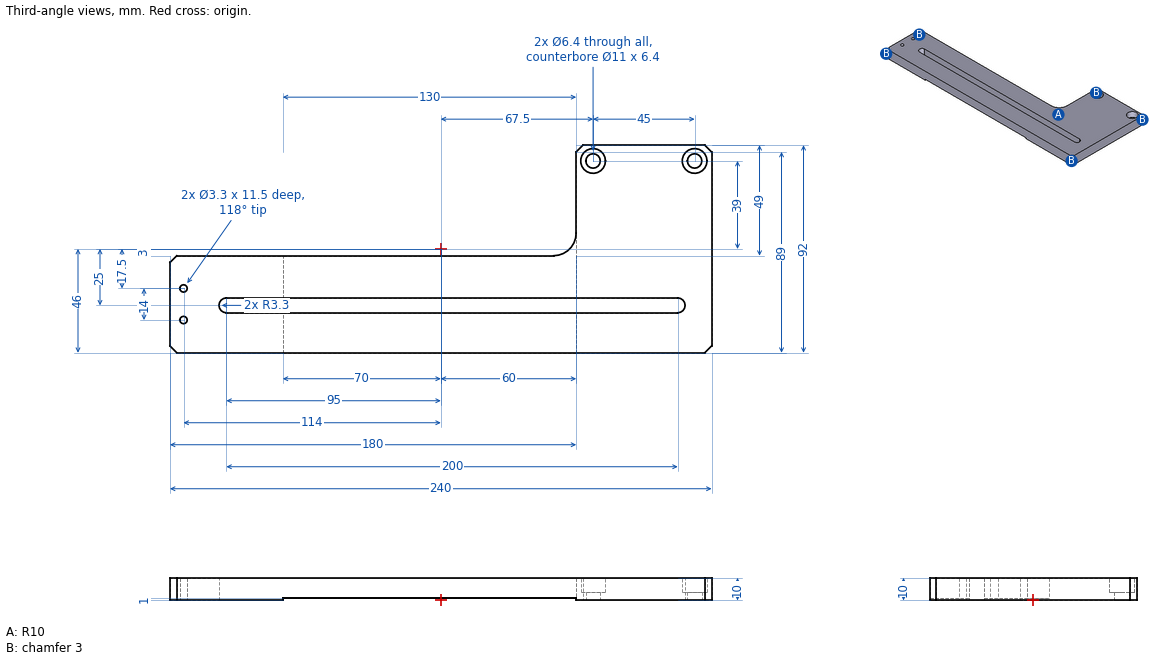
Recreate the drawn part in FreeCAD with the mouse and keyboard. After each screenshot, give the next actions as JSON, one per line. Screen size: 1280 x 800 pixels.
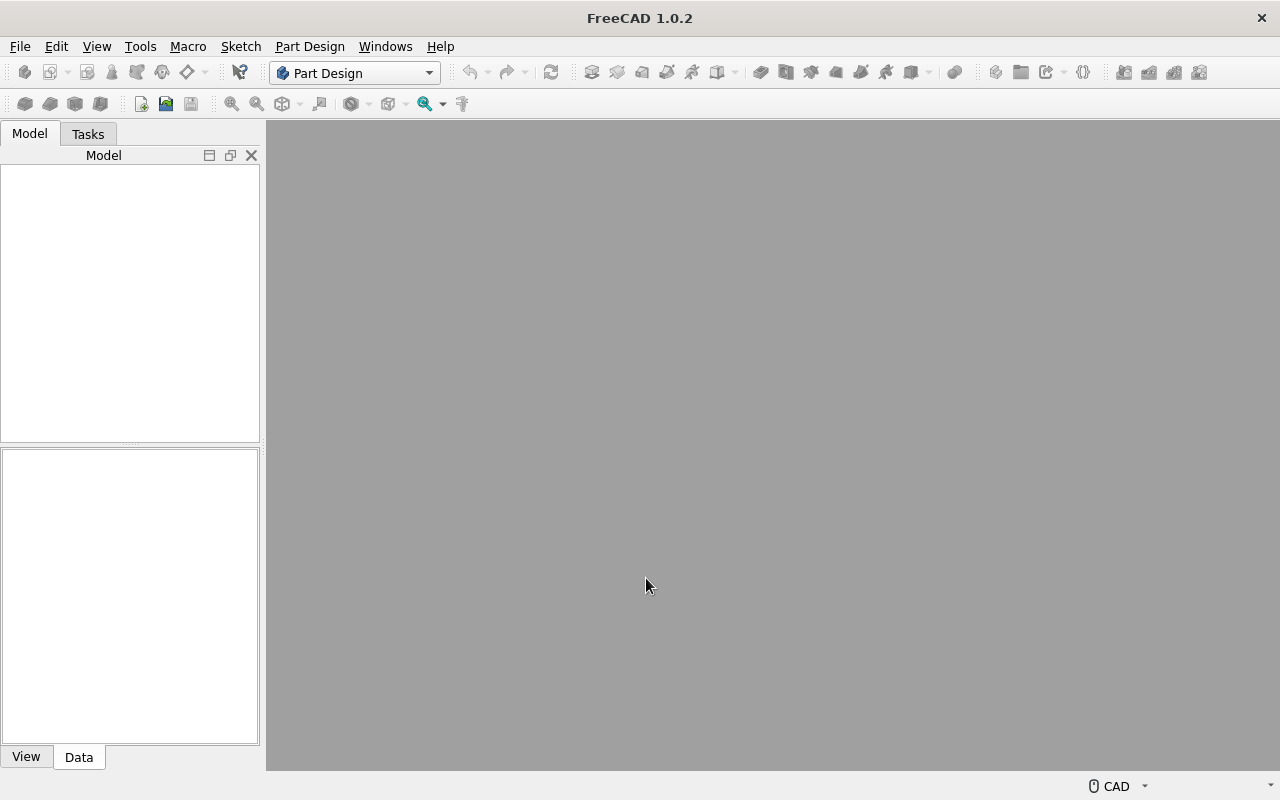
{"action": "left_click", "coordinate": [141, 104]}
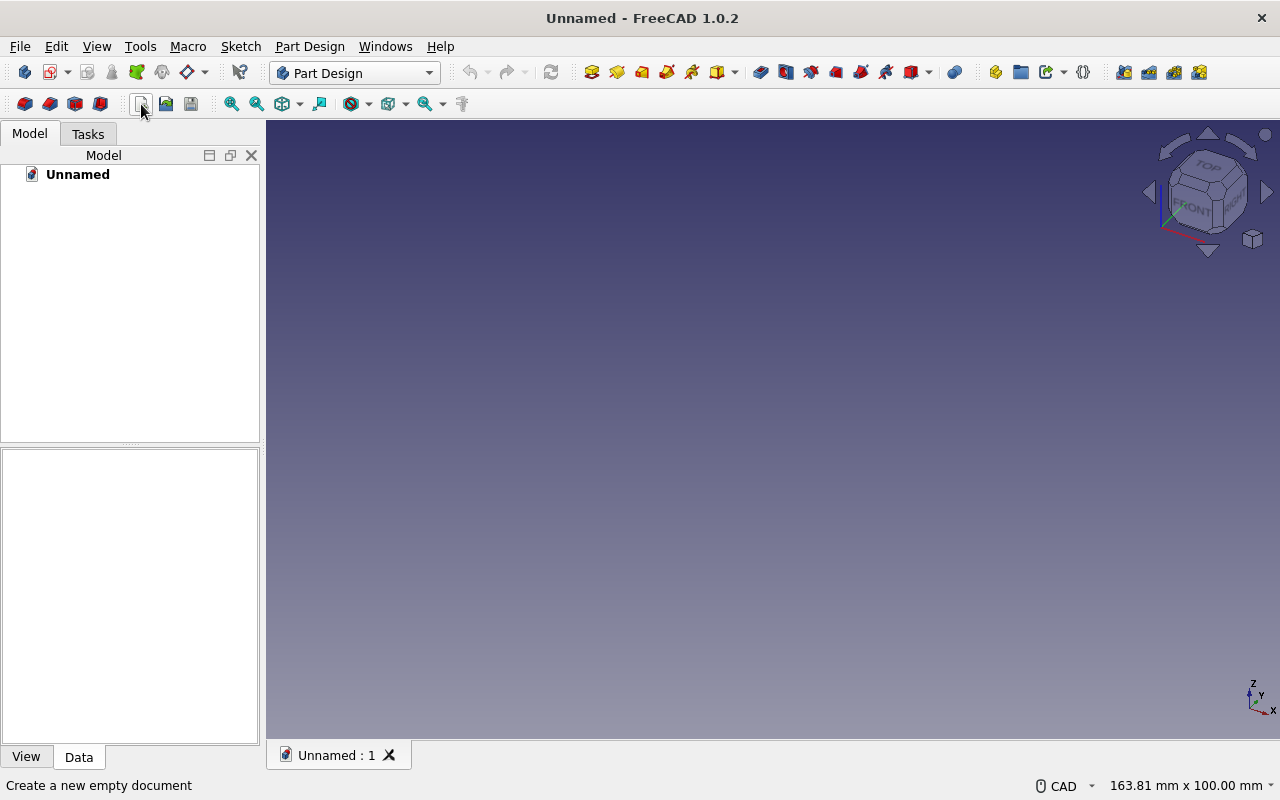
{"action": "left_click", "coordinate": [50, 72]}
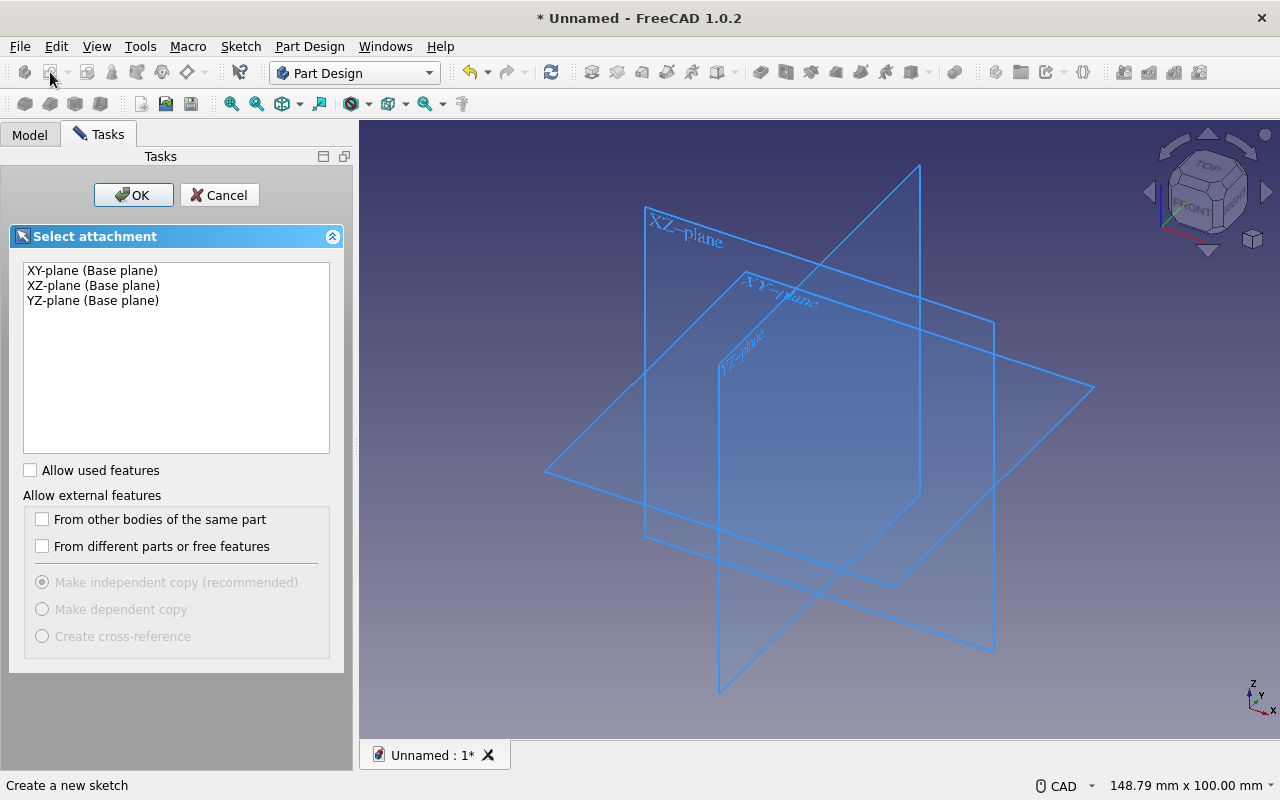
{"action": "left_click", "coordinate": [84, 270]}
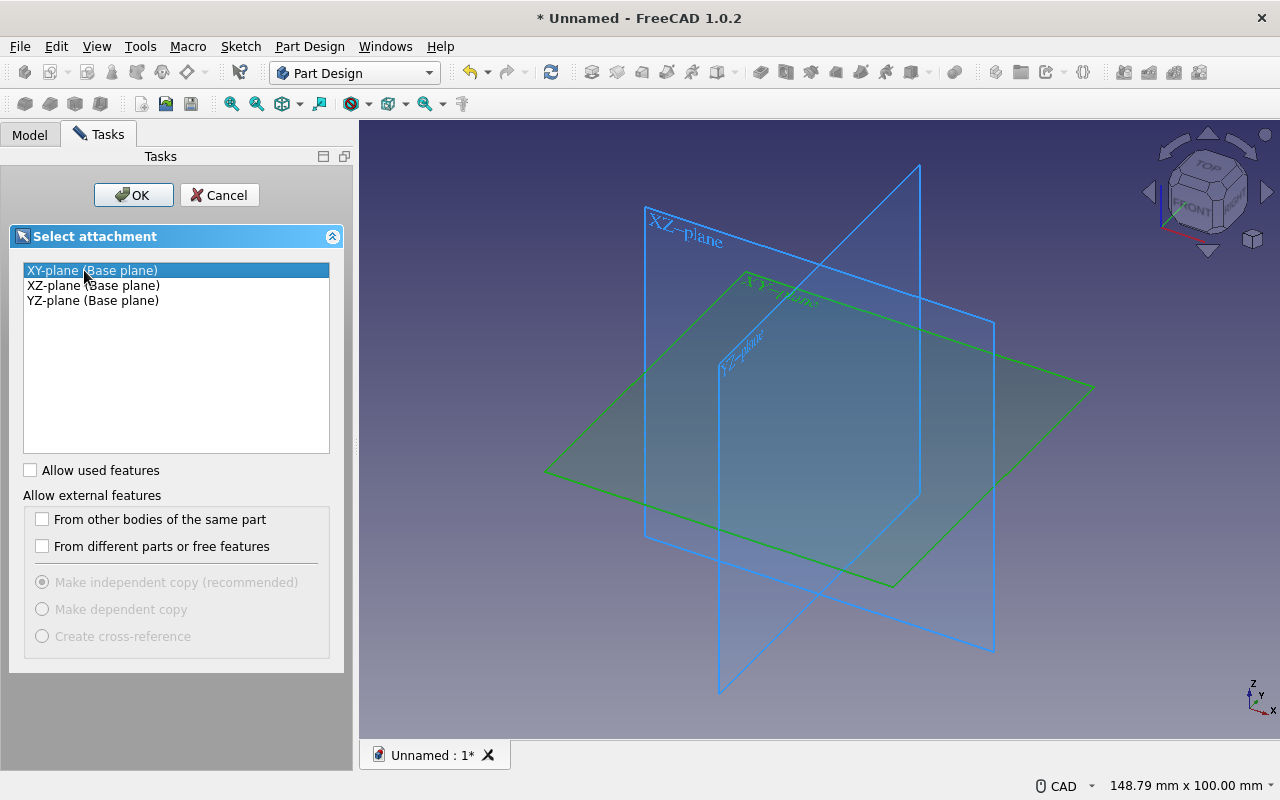
{"action": "left_click", "coordinate": [134, 195]}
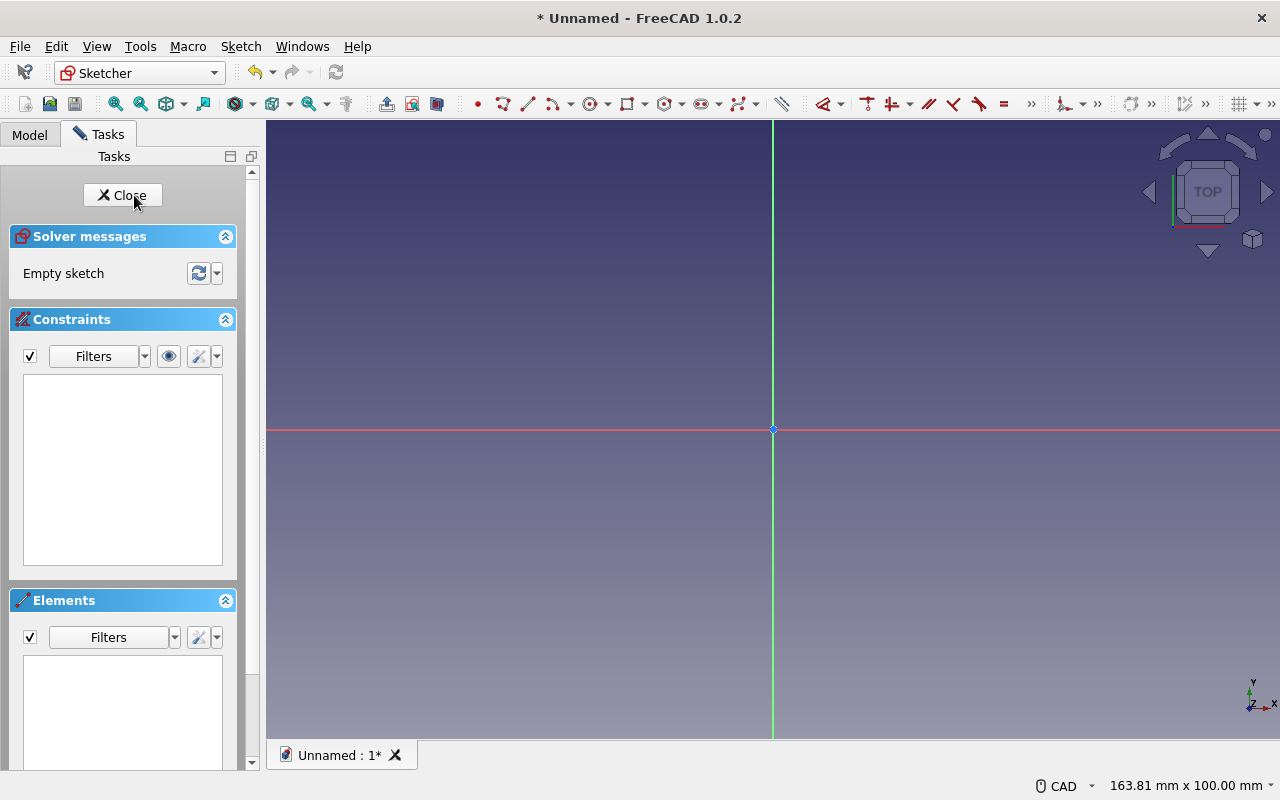
{"action": "scroll", "coordinate": [665, 430], "scroll_direction": "down", "scroll_amount": 5}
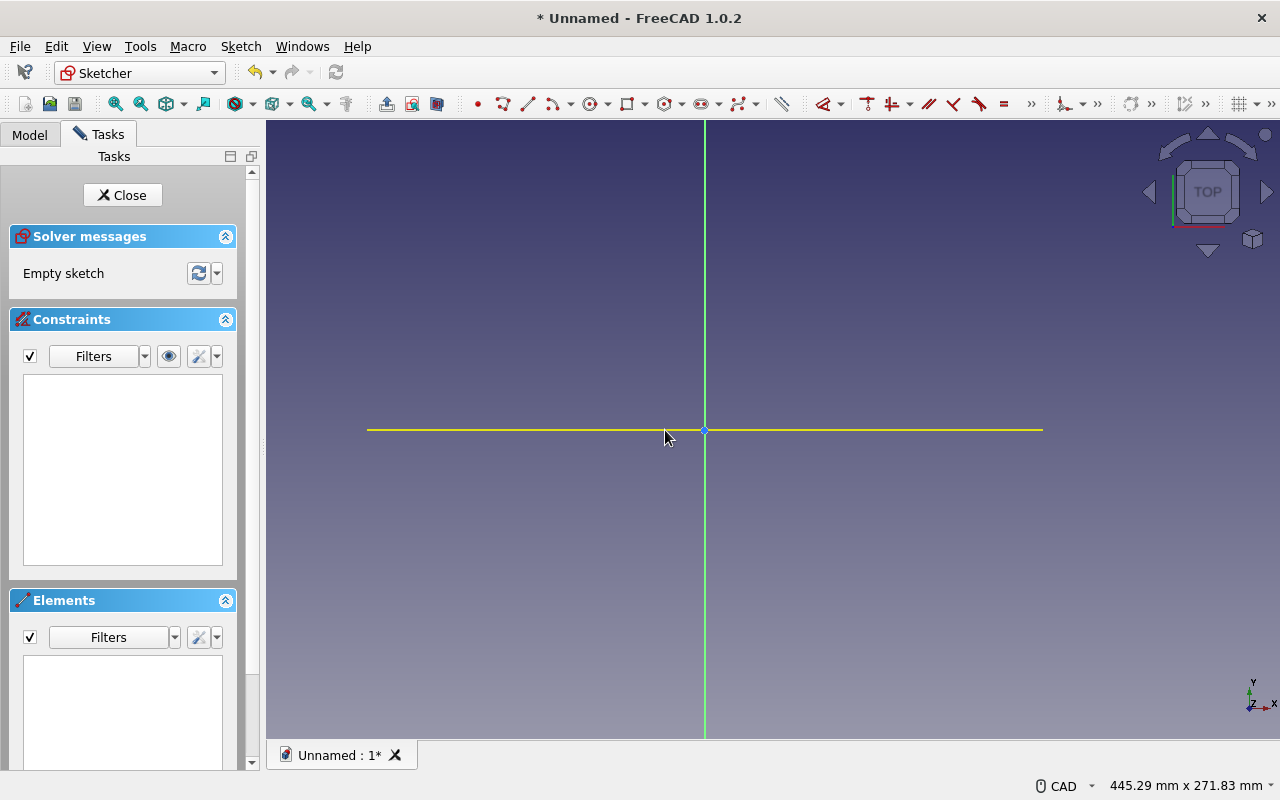
{"action": "key", "text": "g v"}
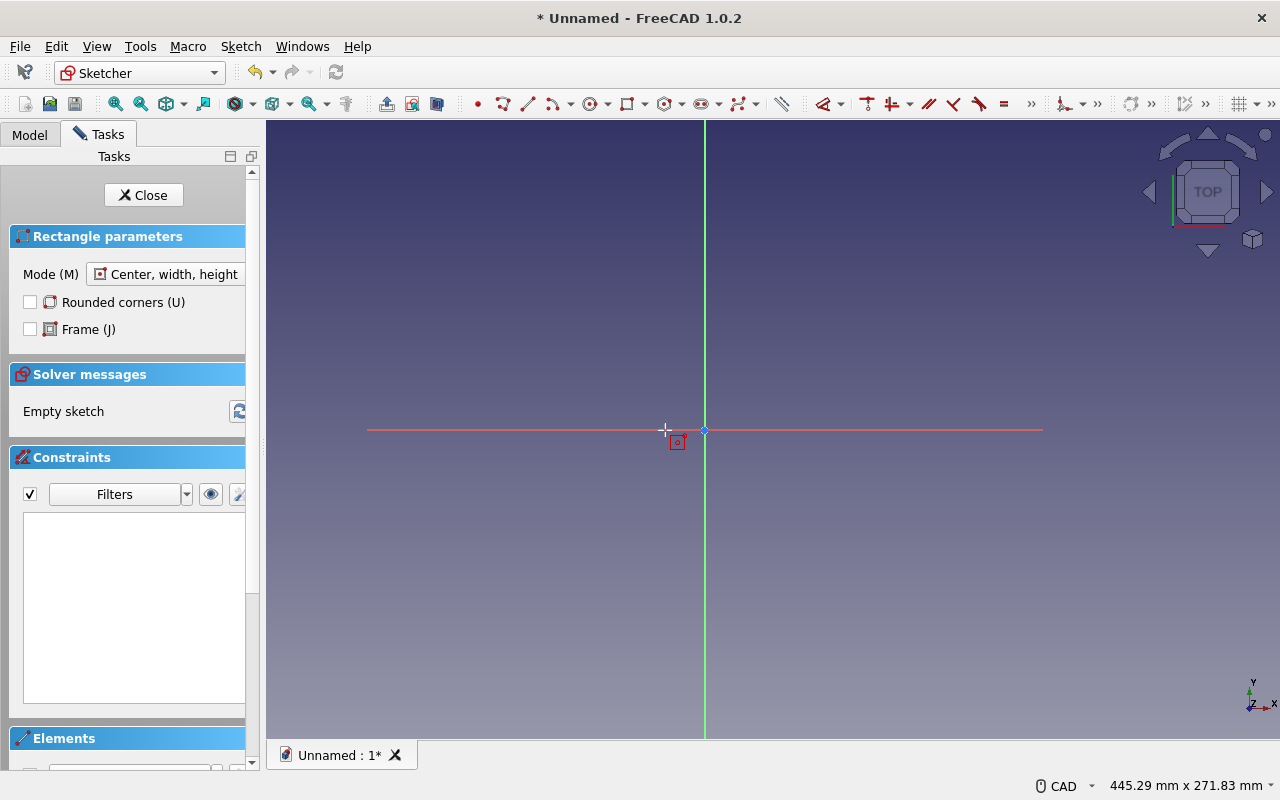
{"action": "left_click", "coordinate": [705, 430]}
{"action": "mouse_move", "coordinate": [978, 325]}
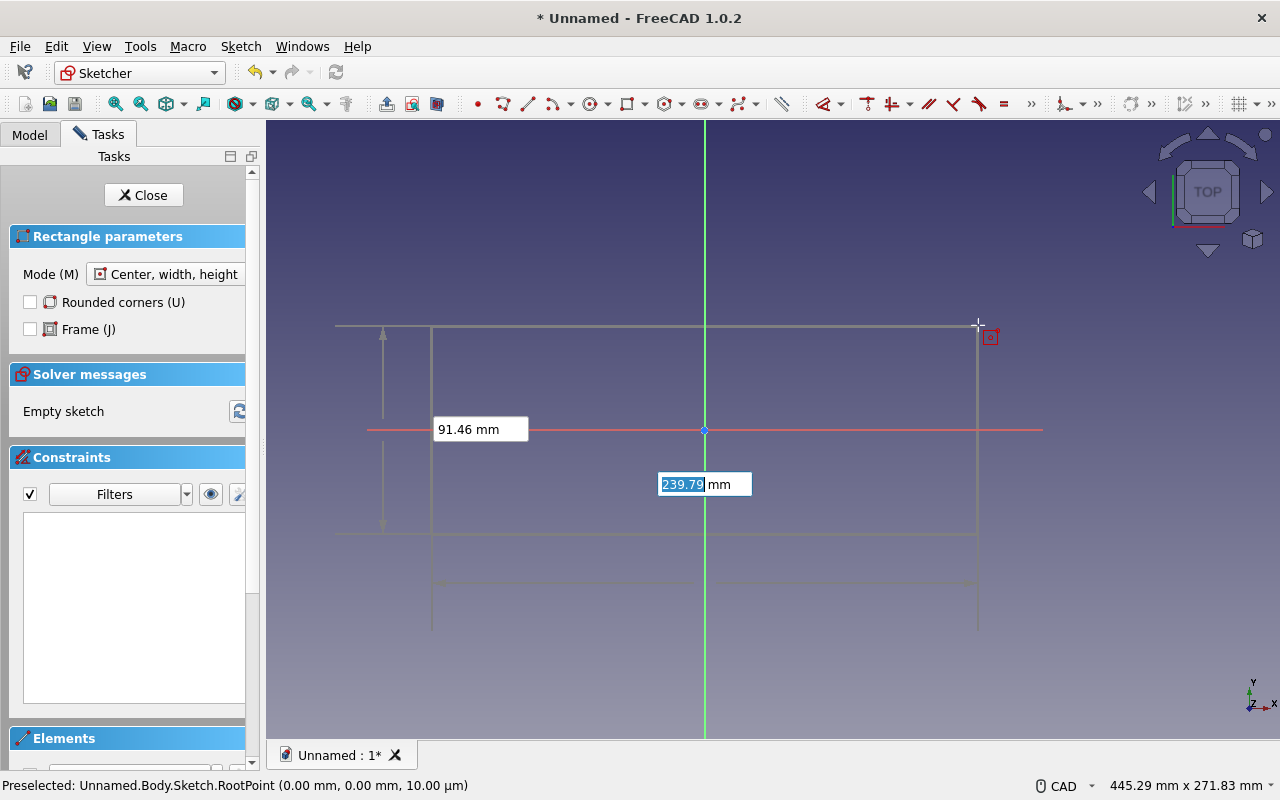
{"action": "type", "text": "240"}
{"action": "key", "text": "Tab"}
{"action": "type", "text": "92"}
{"action": "key", "text": "Return"}
{"action": "key", "text": "Escape"}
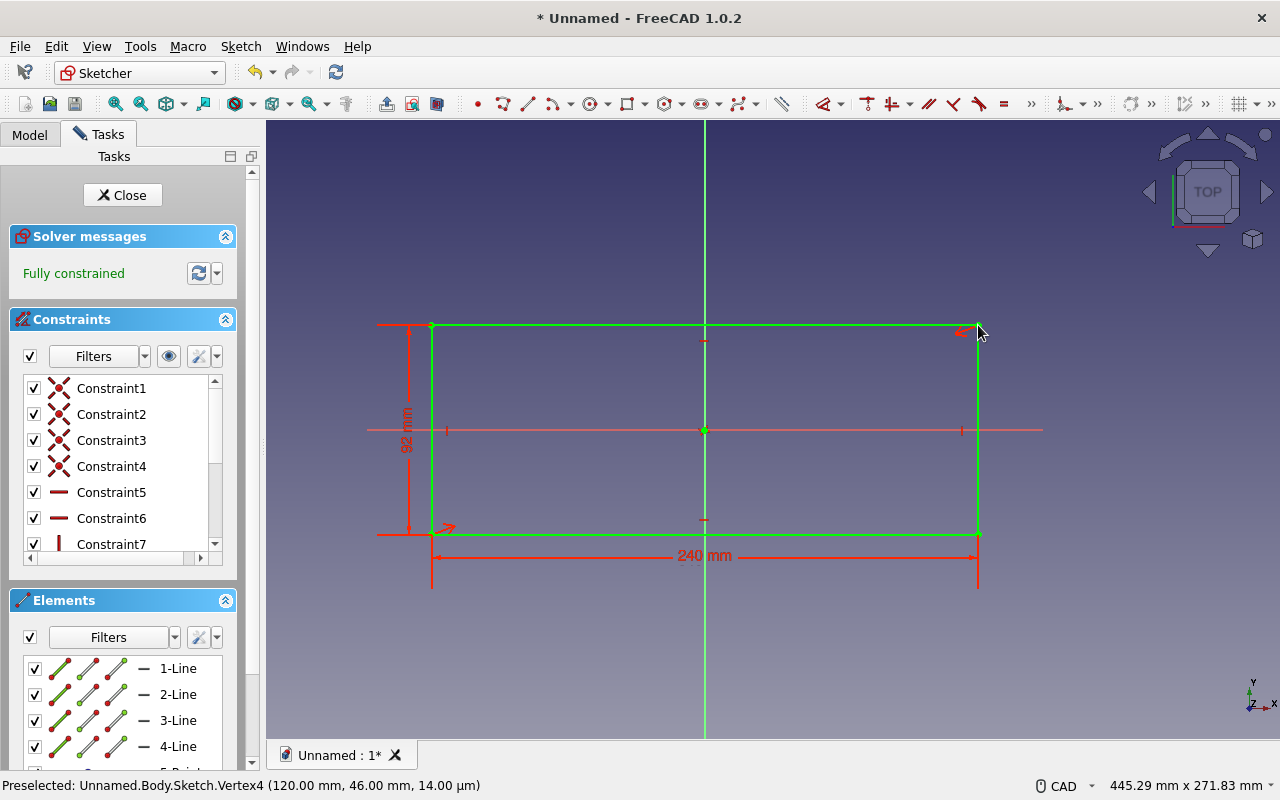
{"action": "left_click", "coordinate": [123, 195]}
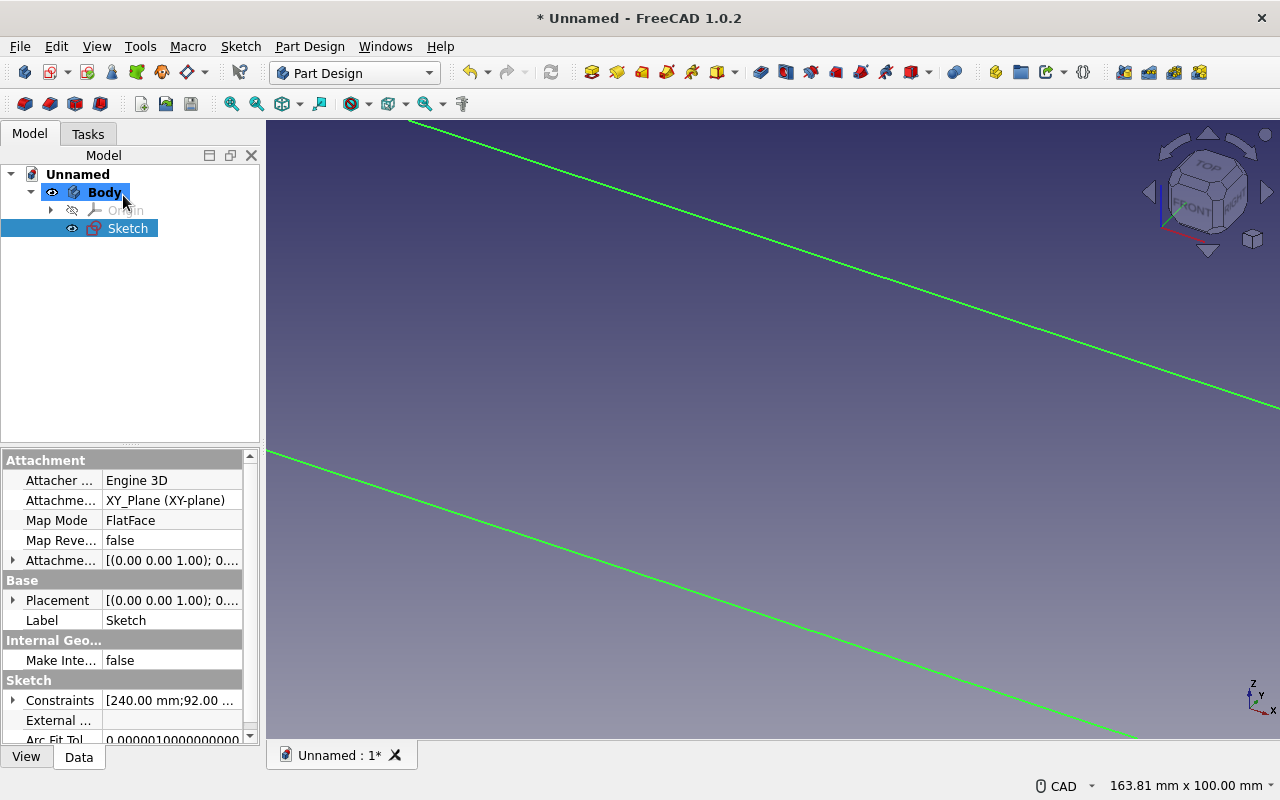
{"action": "left_click", "coordinate": [592, 72]}